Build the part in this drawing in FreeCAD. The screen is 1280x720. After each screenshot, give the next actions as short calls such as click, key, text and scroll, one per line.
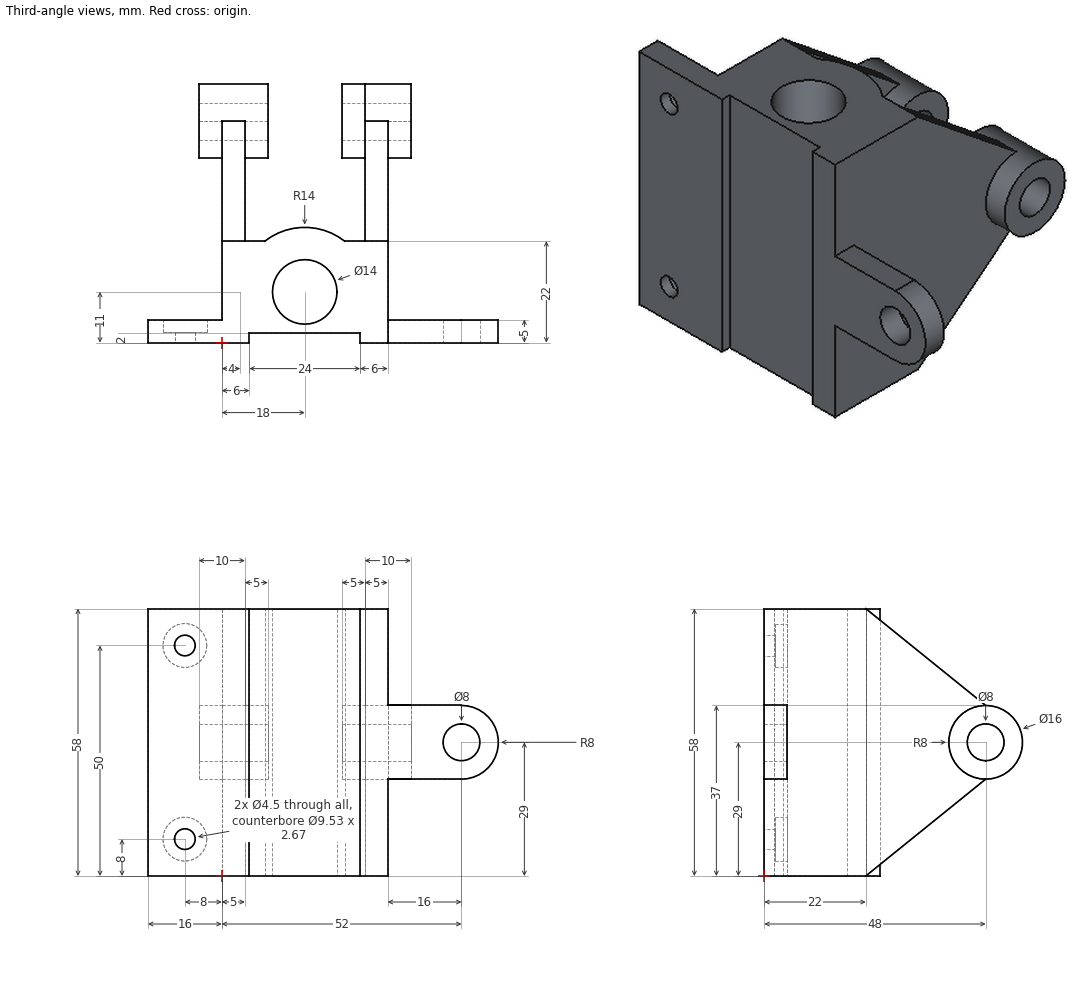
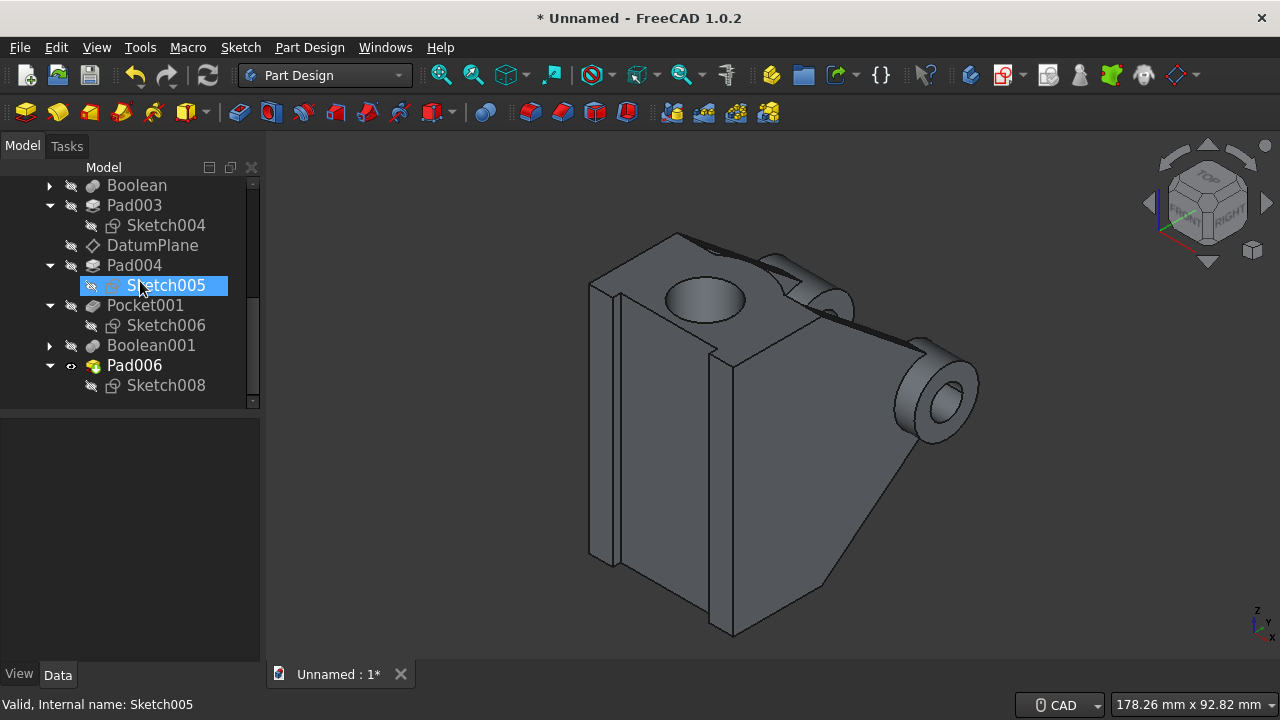
scroll(140, 281, up, 15)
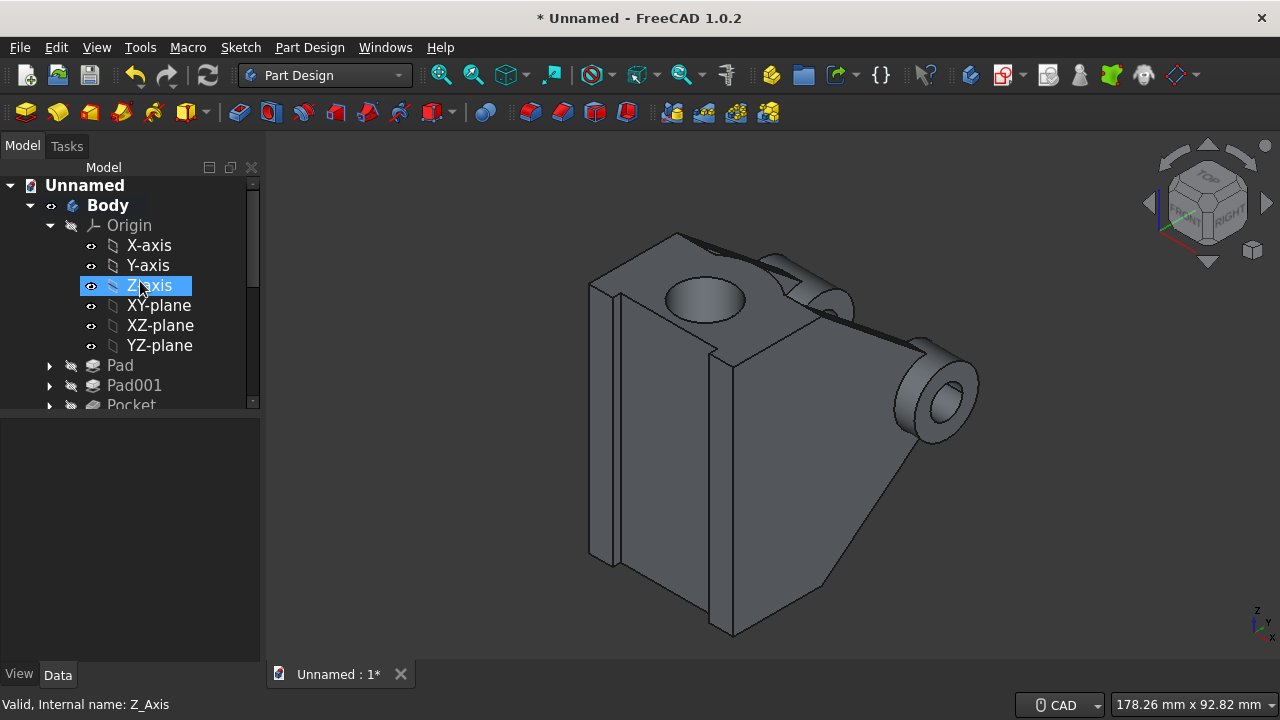
click(136, 346)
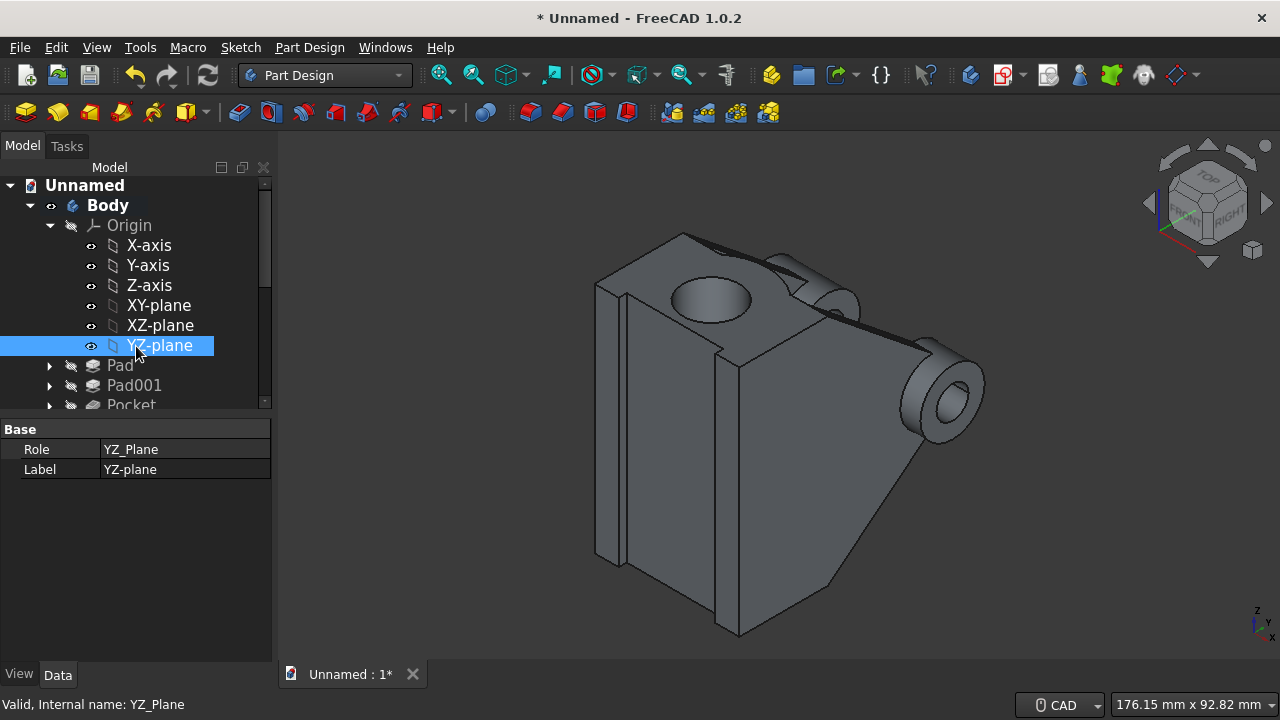
click(1176, 76)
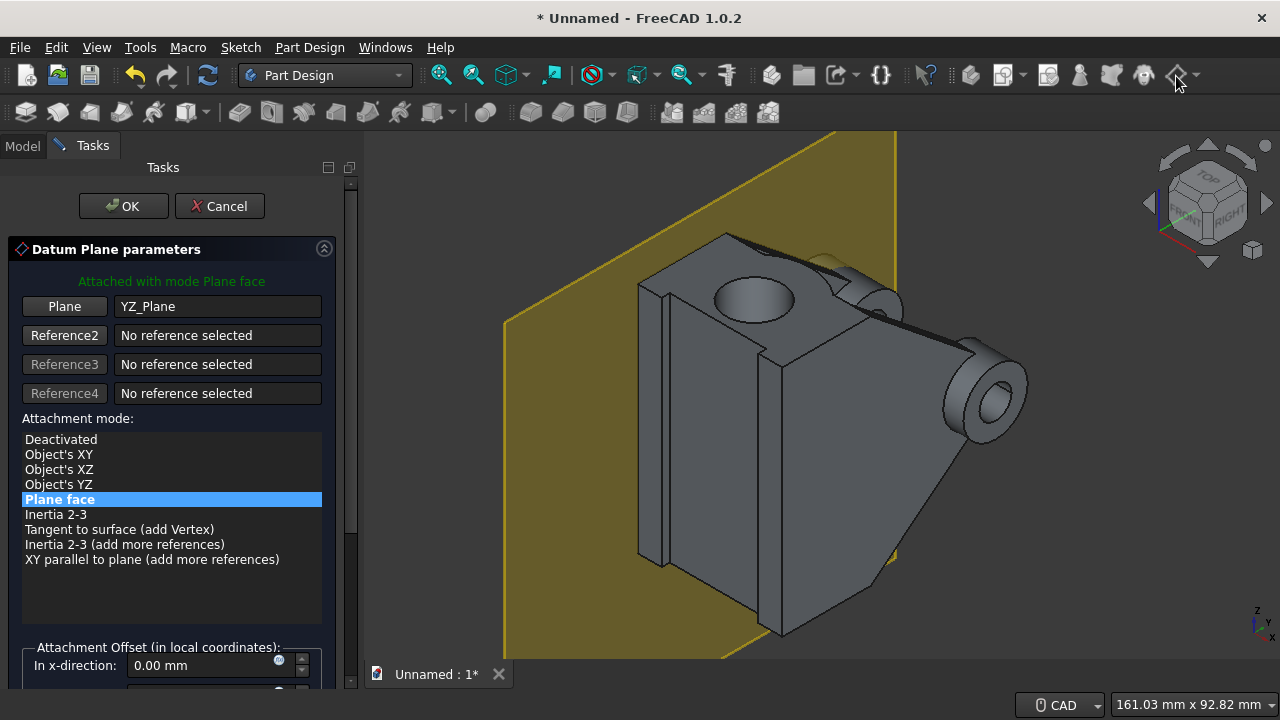
scroll(351, 432, down, 2)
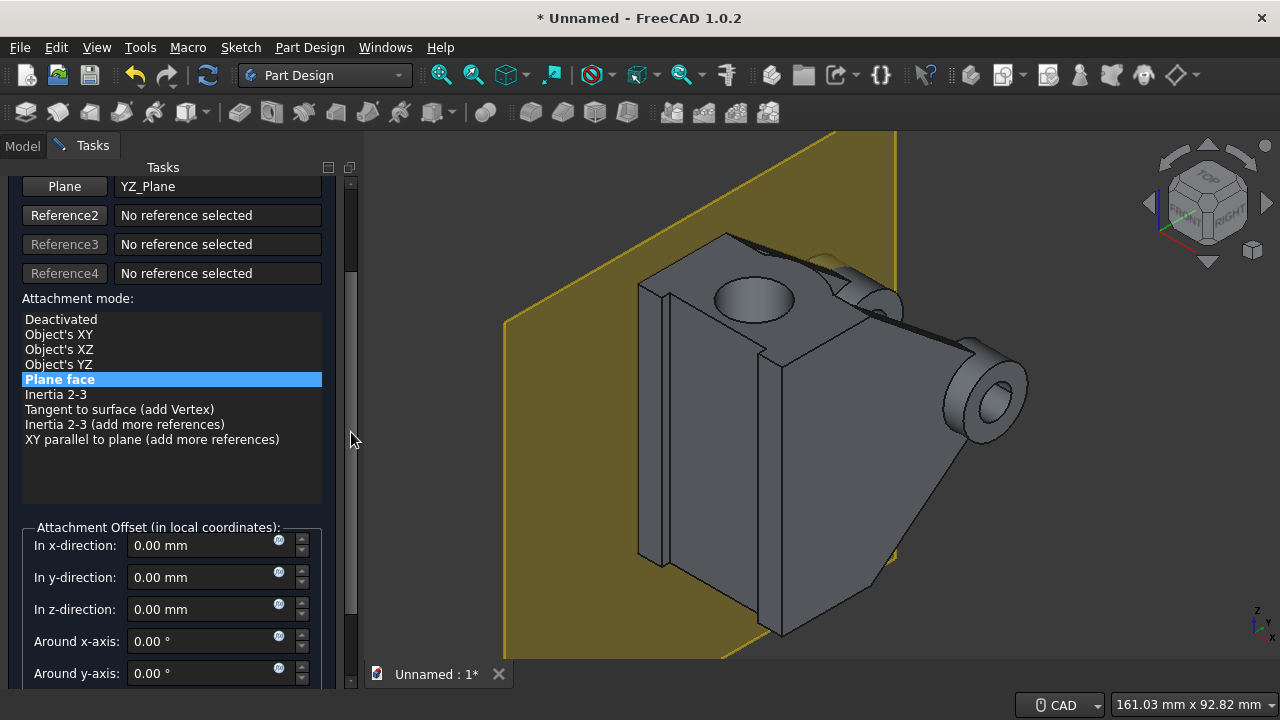
triple_click(210, 609)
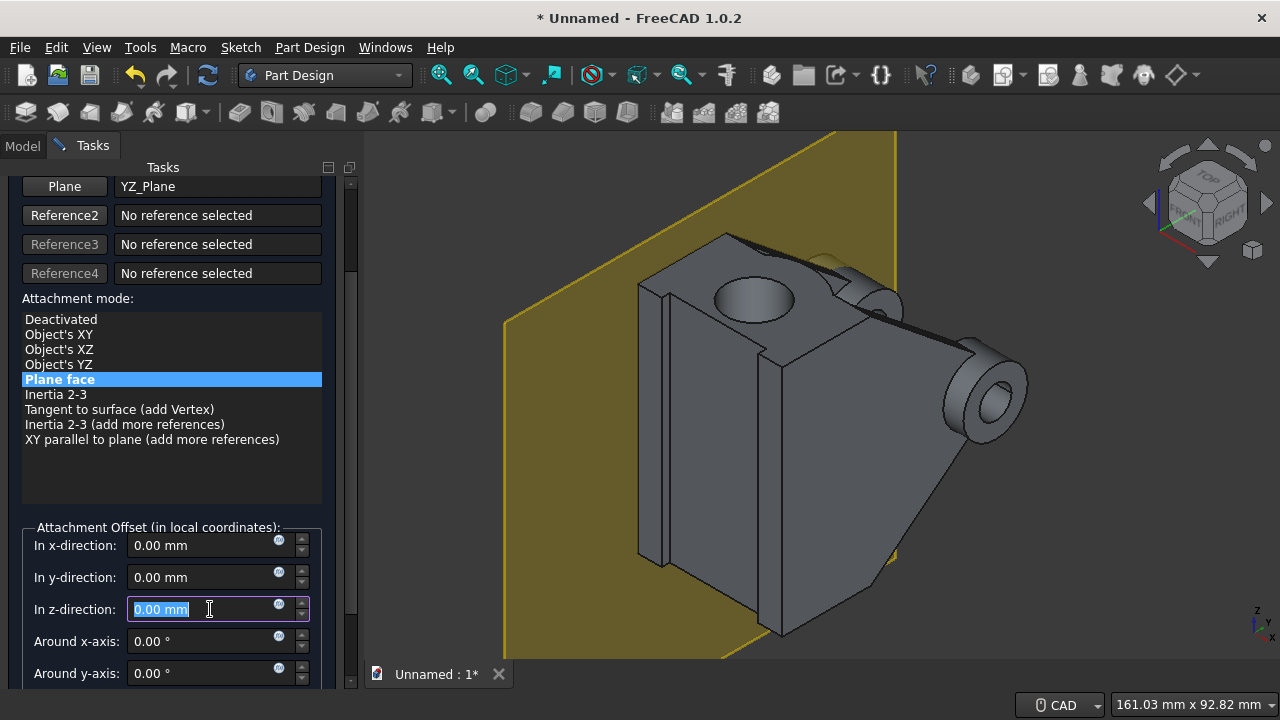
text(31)
key(Tab)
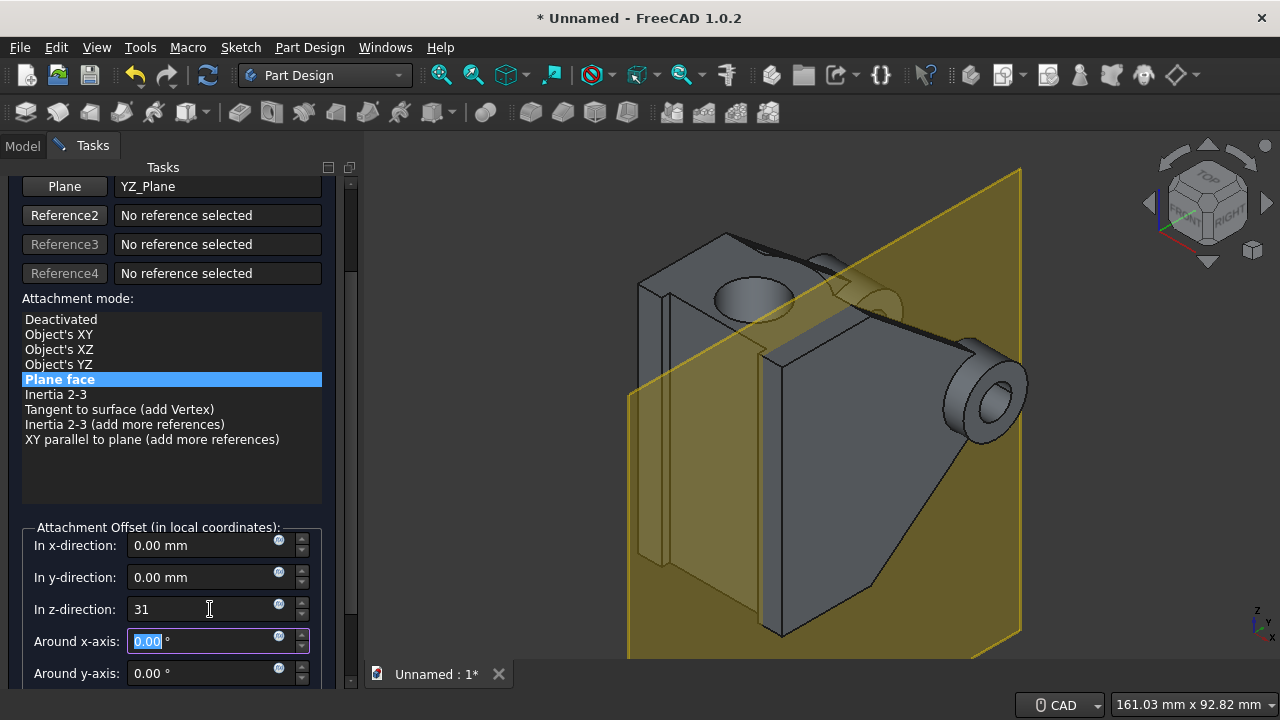
scroll(351, 432, up, 3)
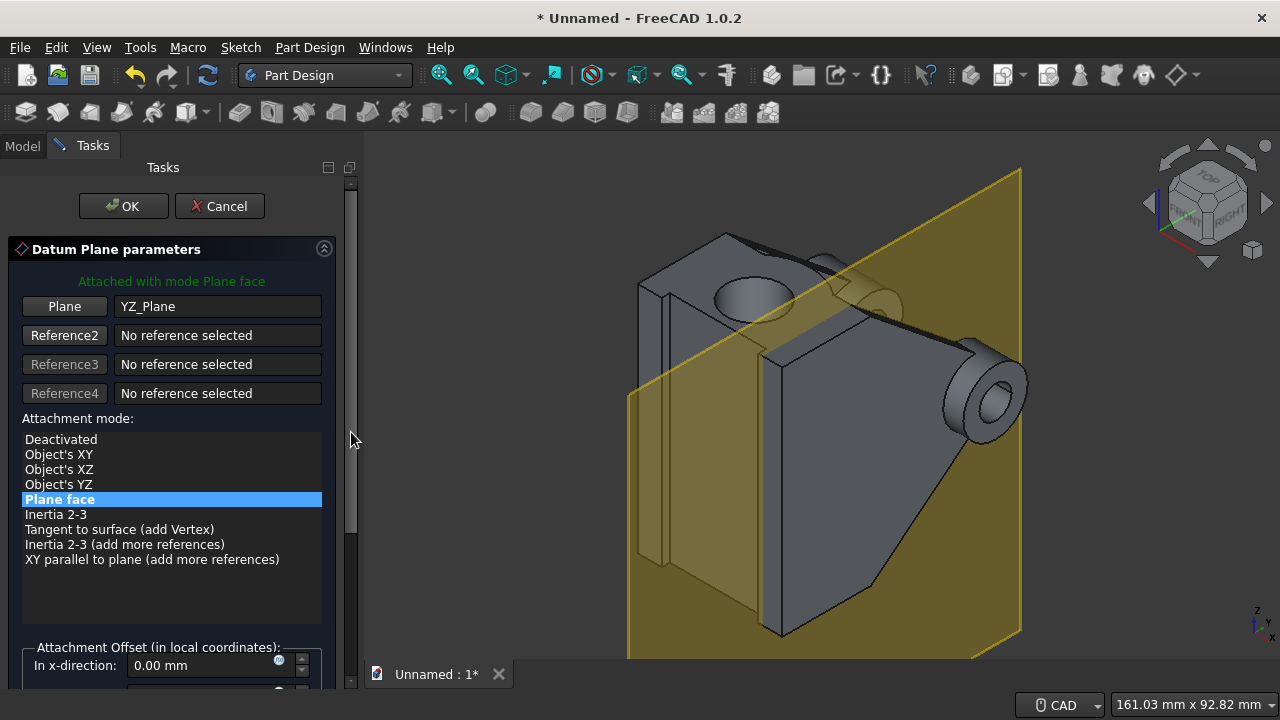
click(124, 206)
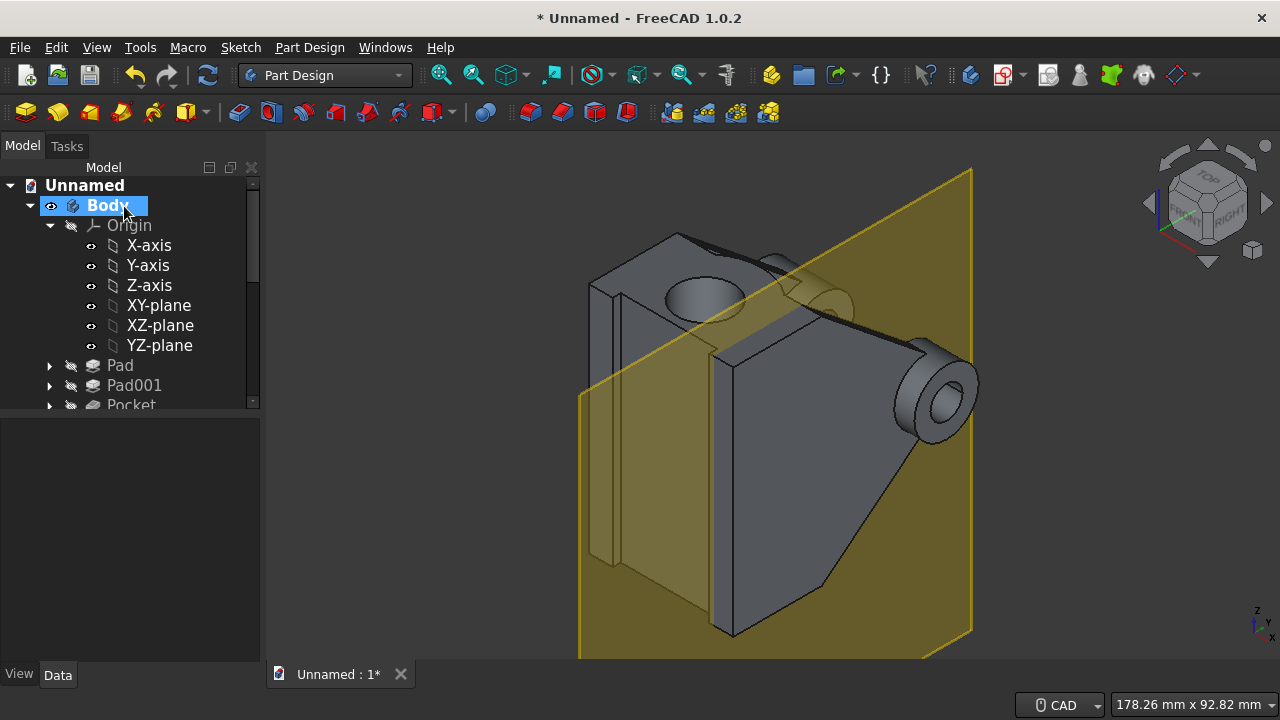
scroll(100, 301, down, 3)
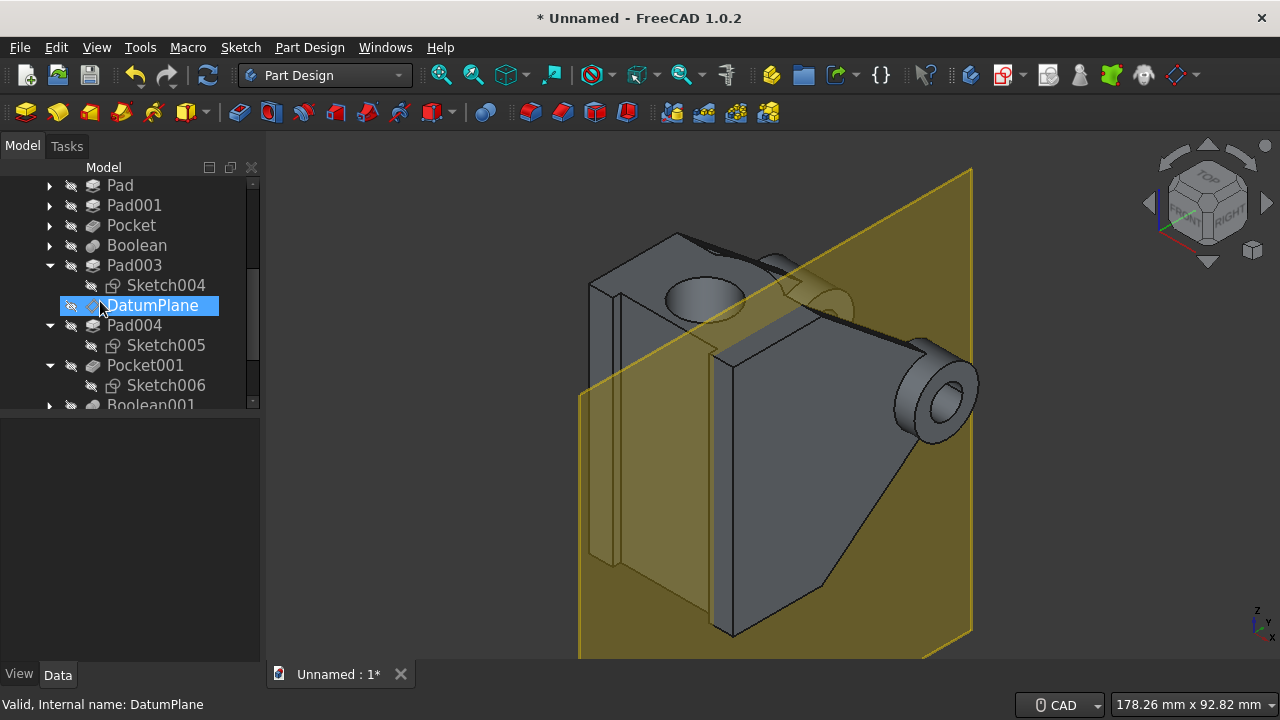
scroll(140, 301, up, 15)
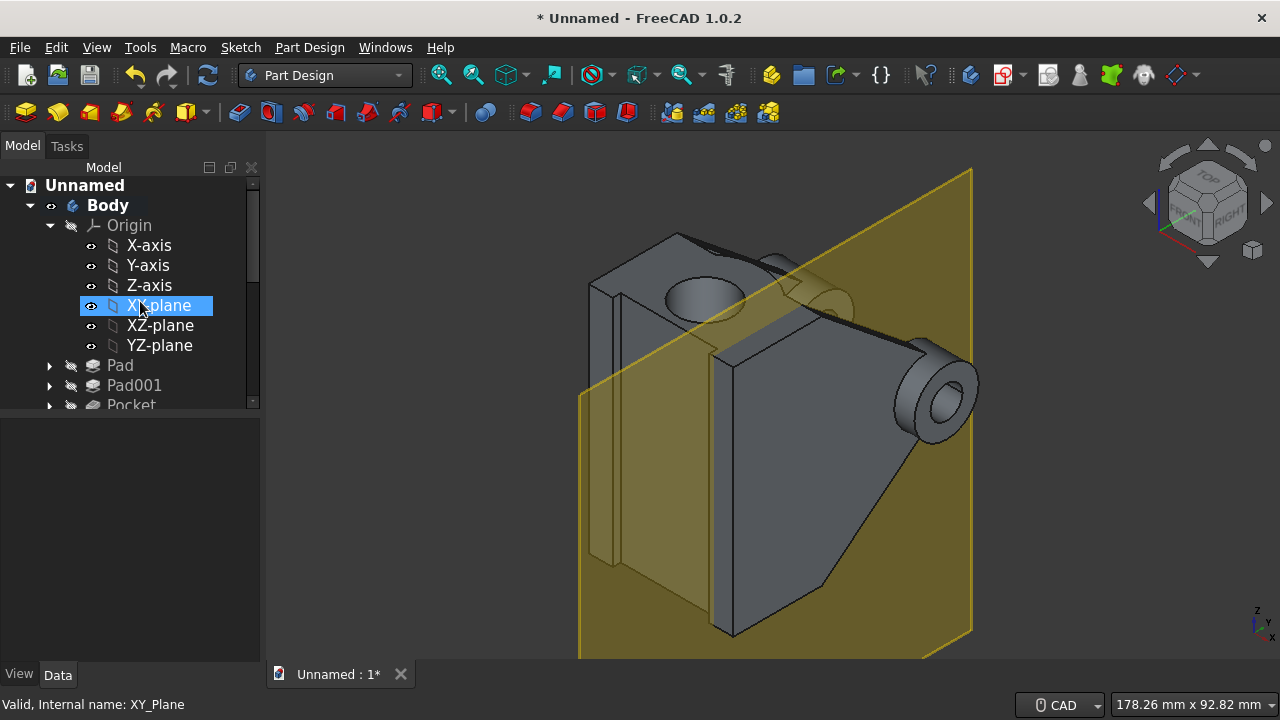
scroll(100, 301, down, 6)